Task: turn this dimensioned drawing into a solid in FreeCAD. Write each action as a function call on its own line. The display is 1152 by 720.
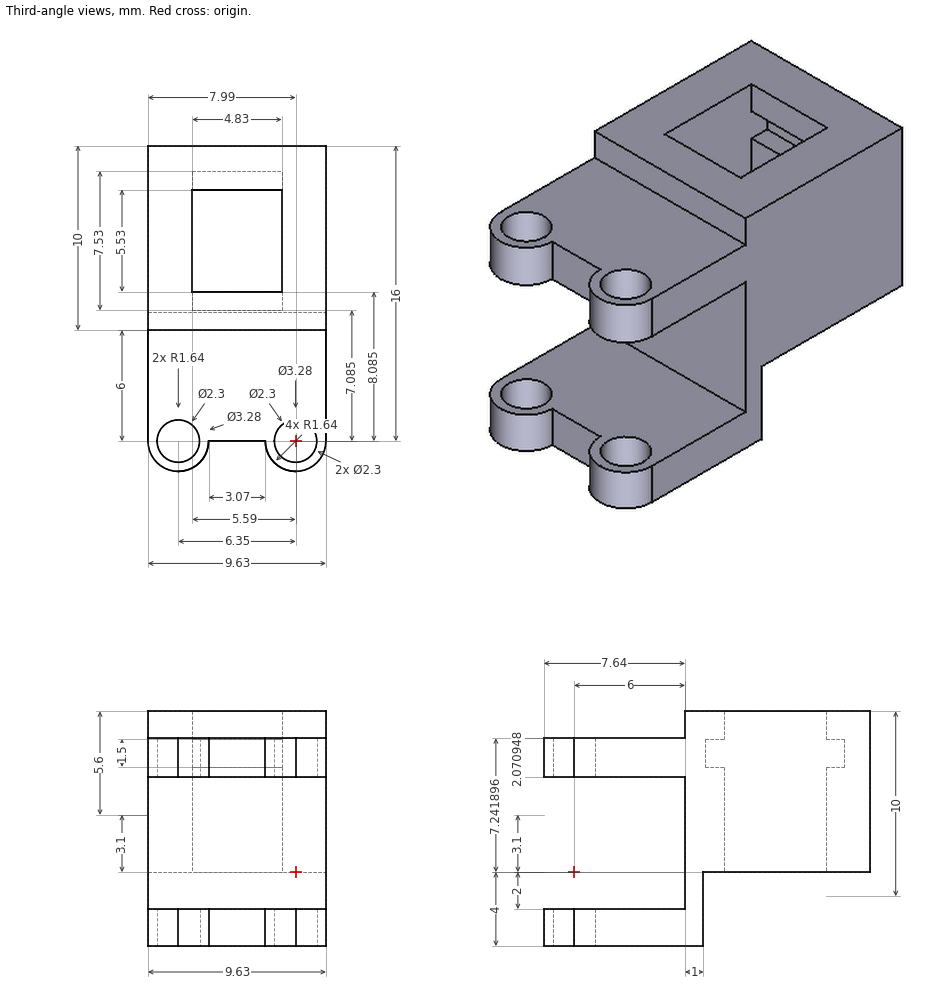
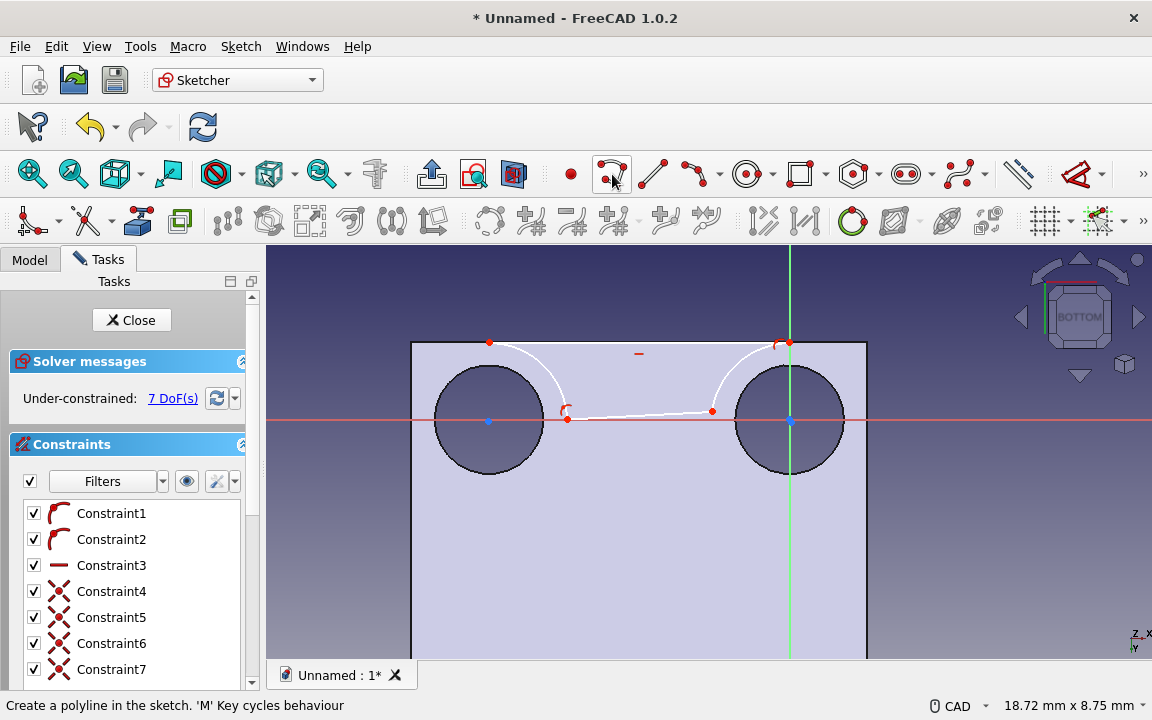
click(867, 420)
click(867, 342)
click(790, 343)
right_click(867, 342)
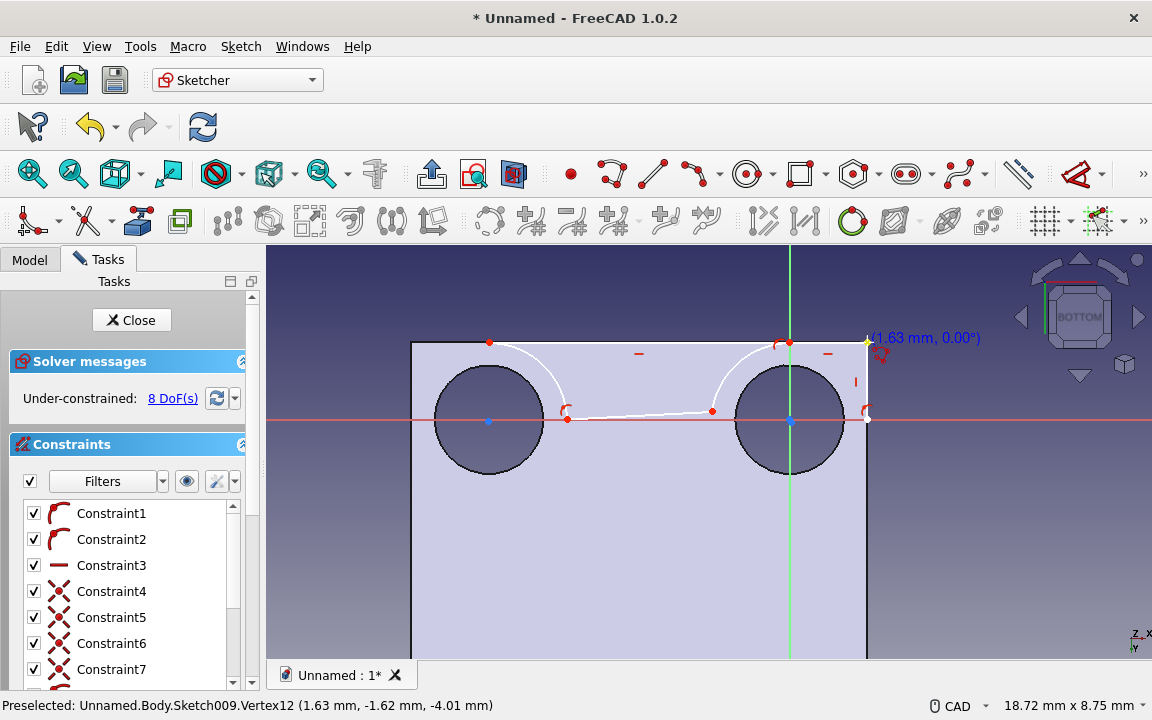
click(694, 174)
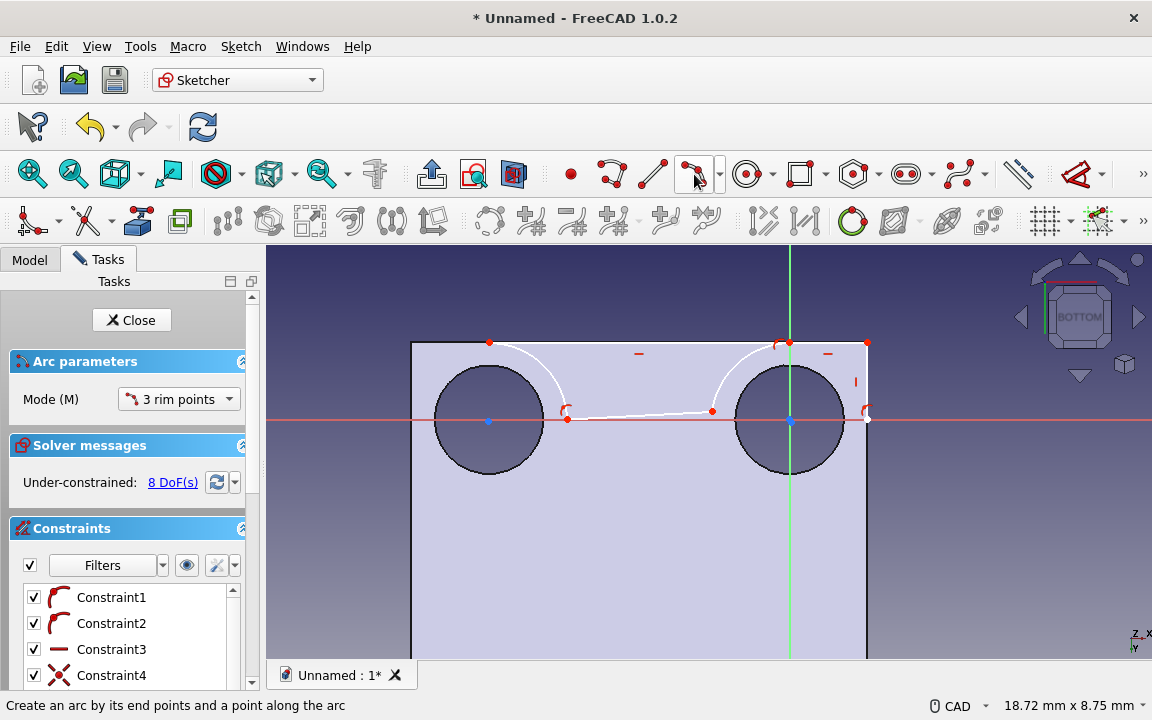
click(790, 343)
click(867, 420)
click(845, 365)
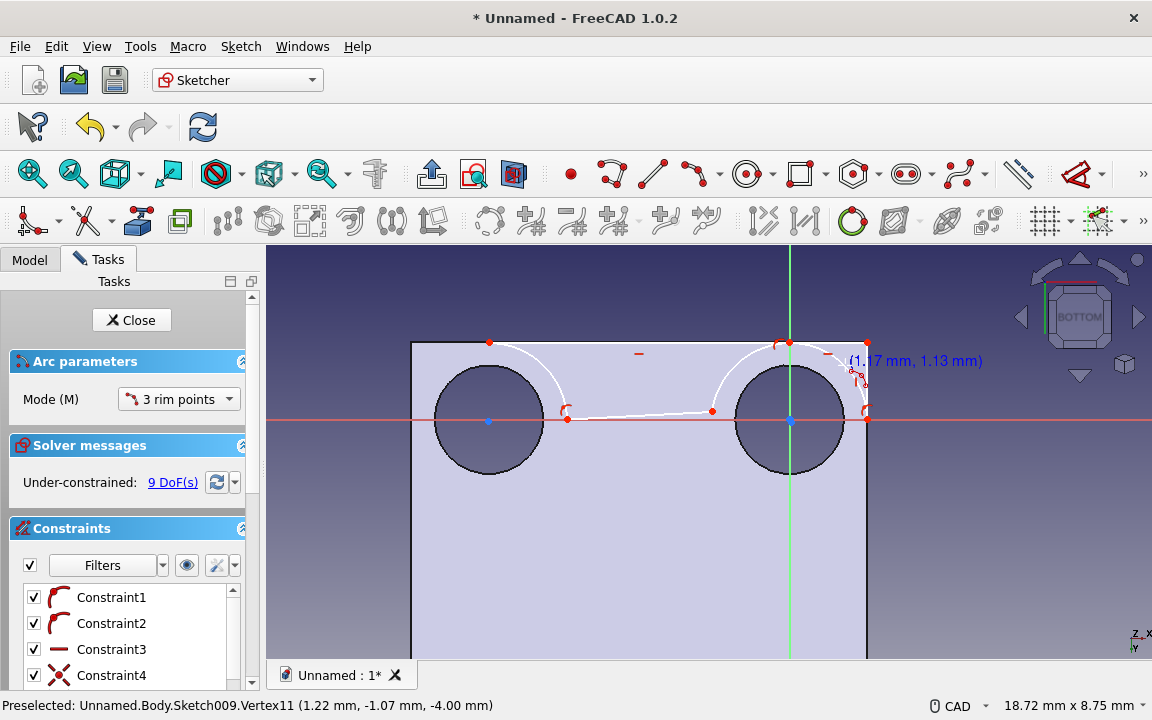
click(612, 174)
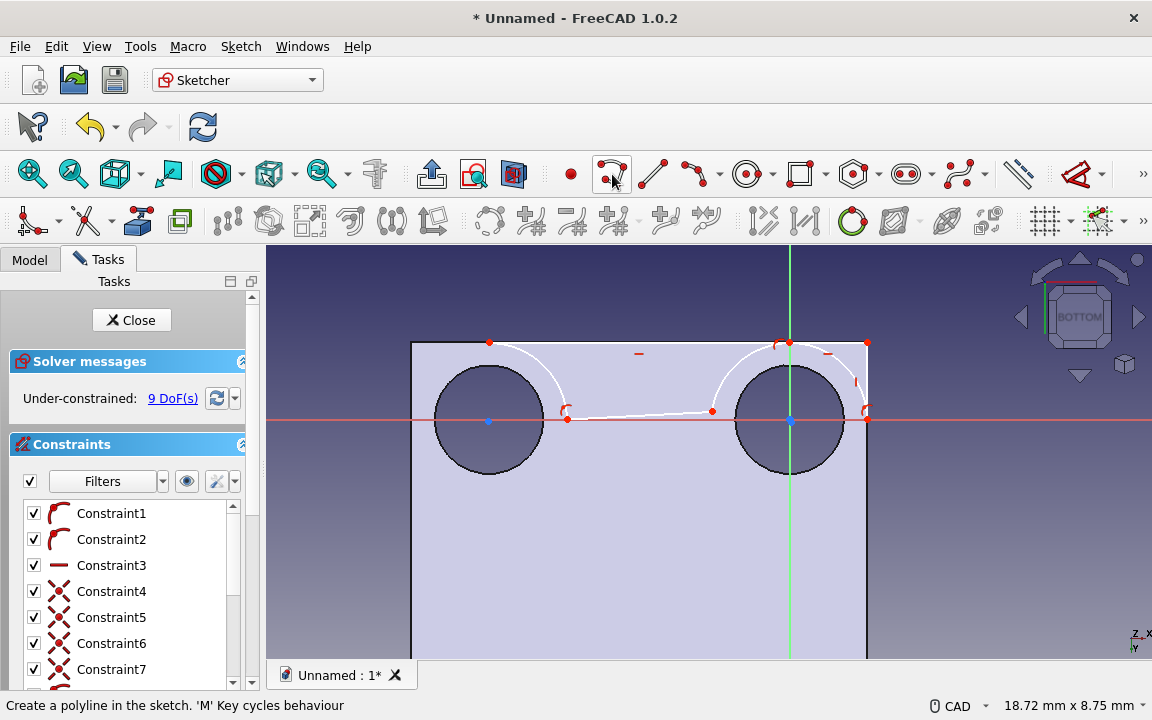
click(489, 343)
click(411, 342)
click(411, 420)
right_click(411, 420)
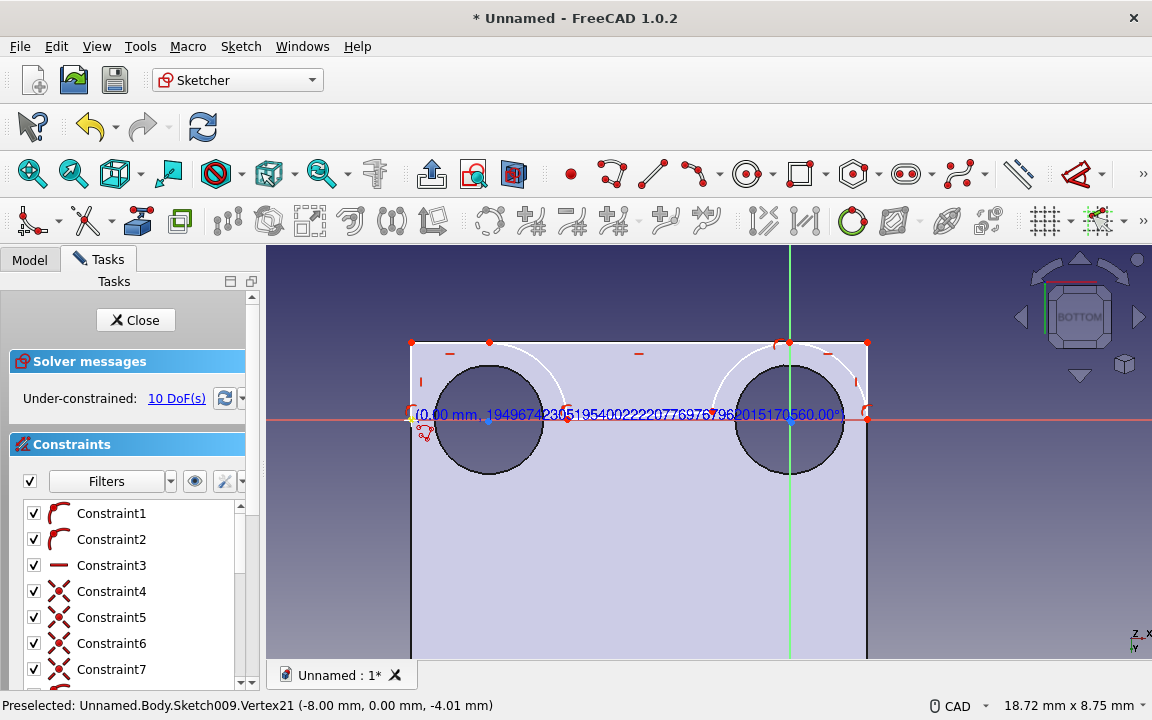
click(694, 174)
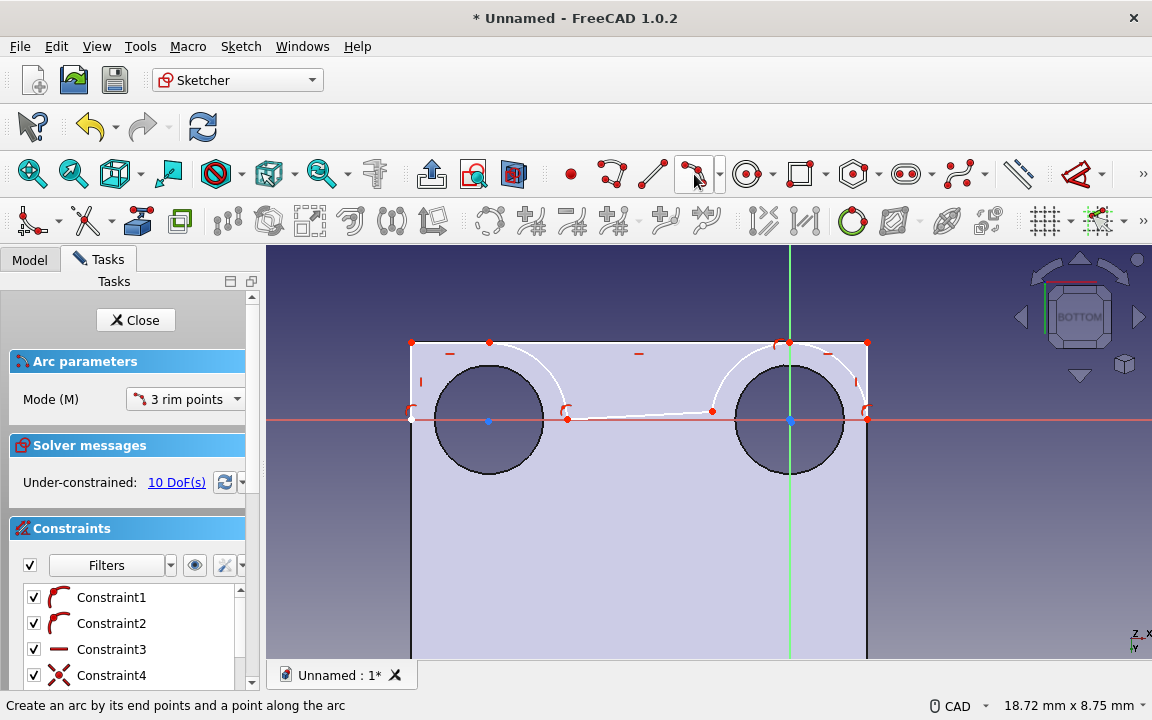
click(411, 420)
click(489, 343)
click(434, 365)
key(Escape)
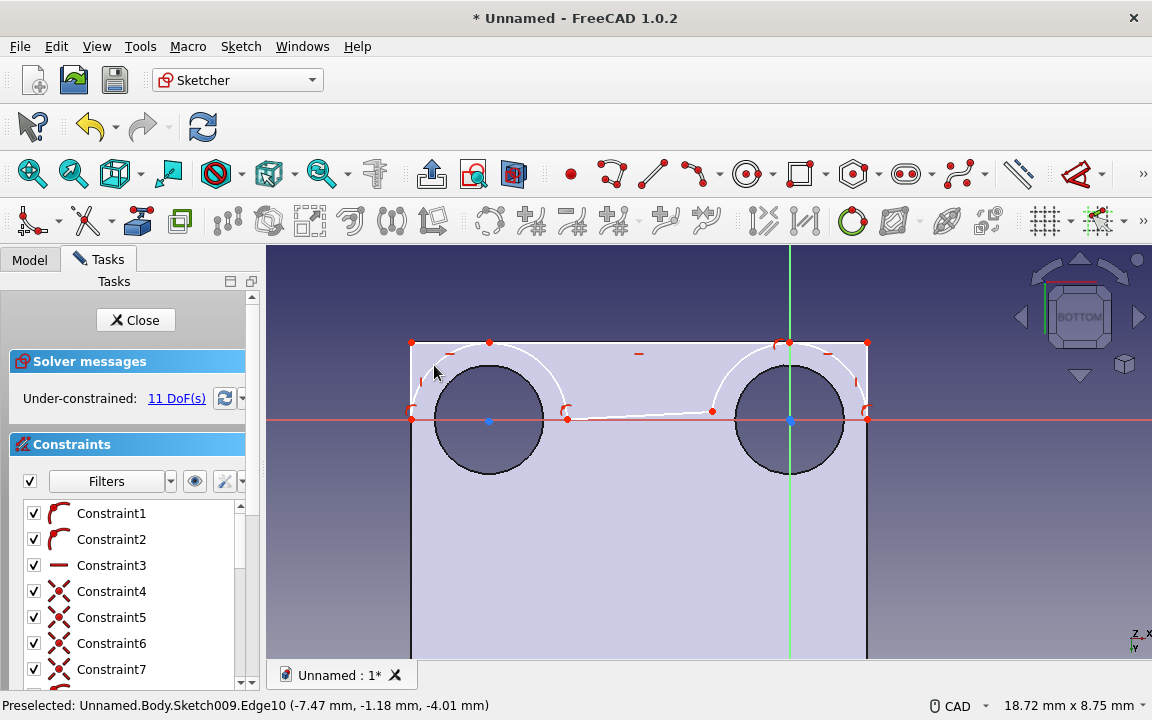
click(699, 343)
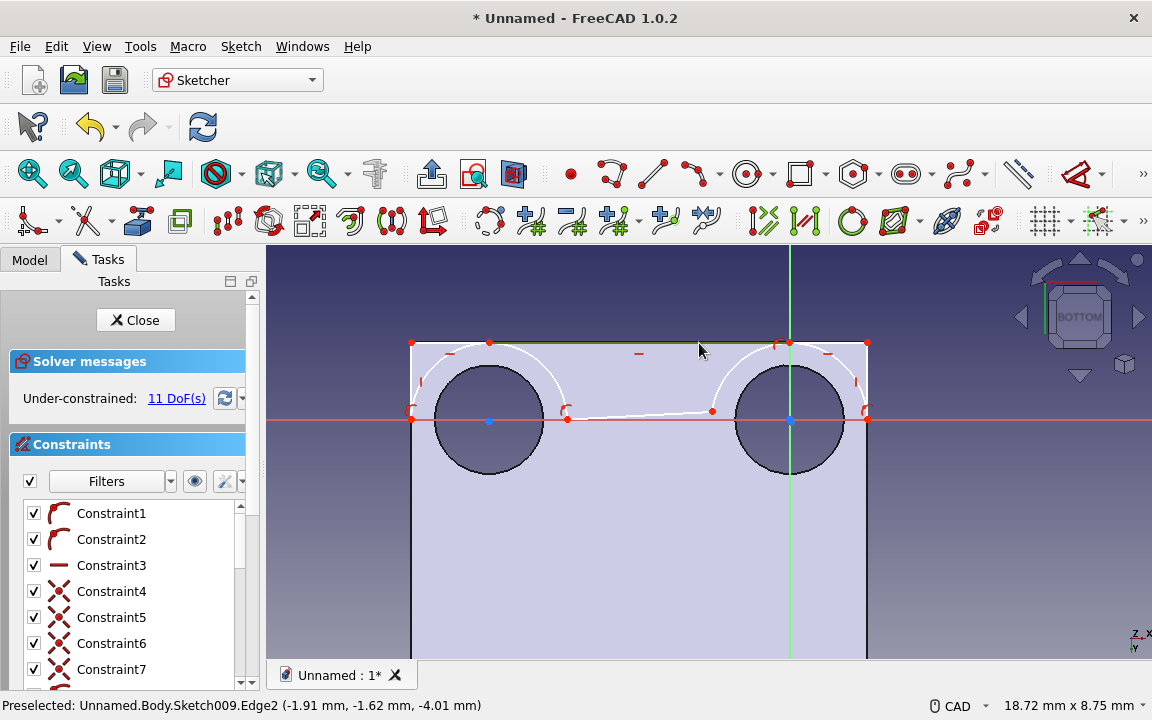
click(723, 380)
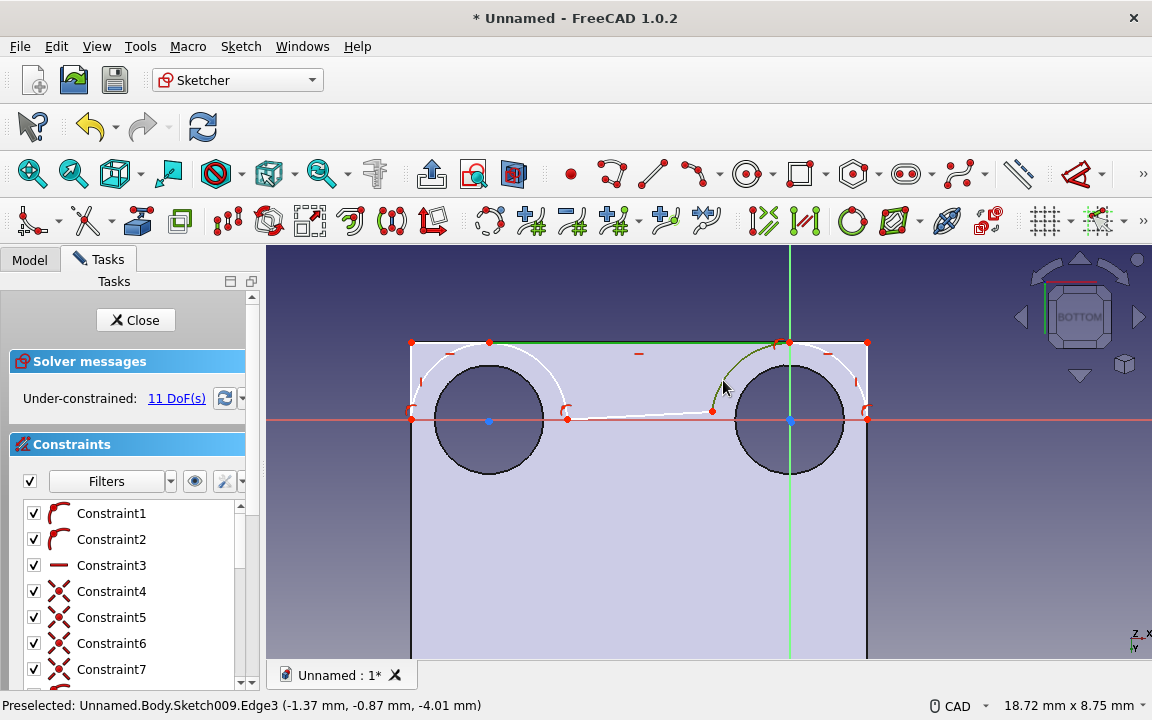
key(t)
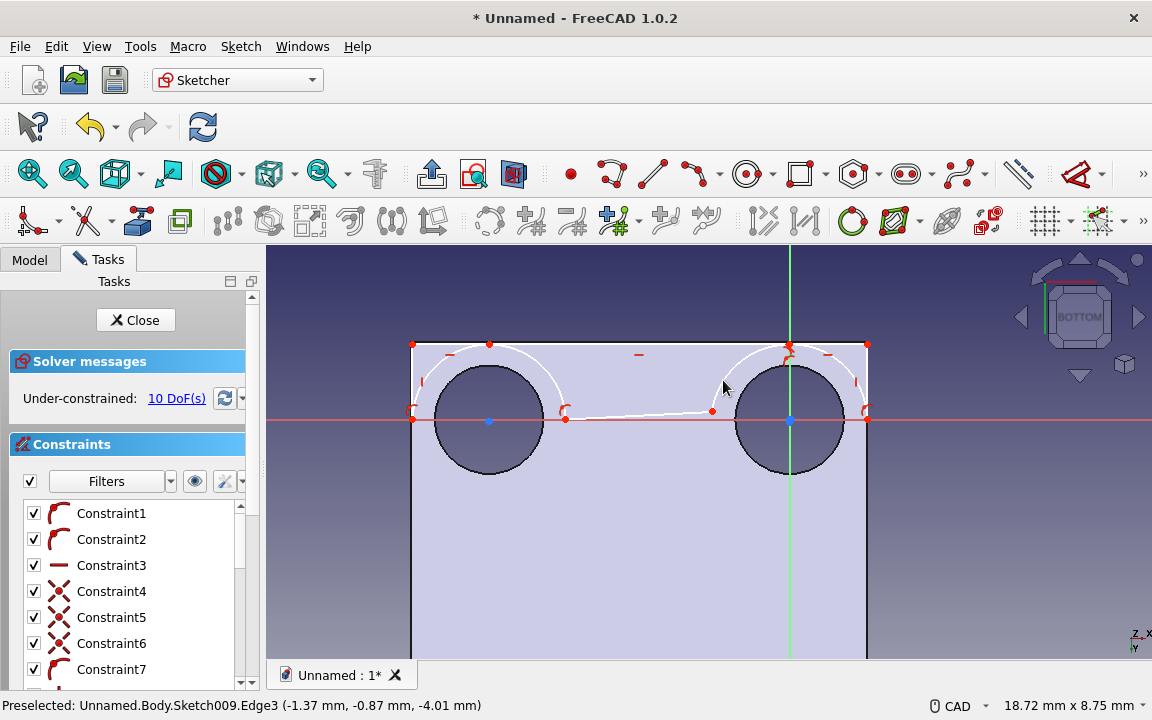
click(699, 344)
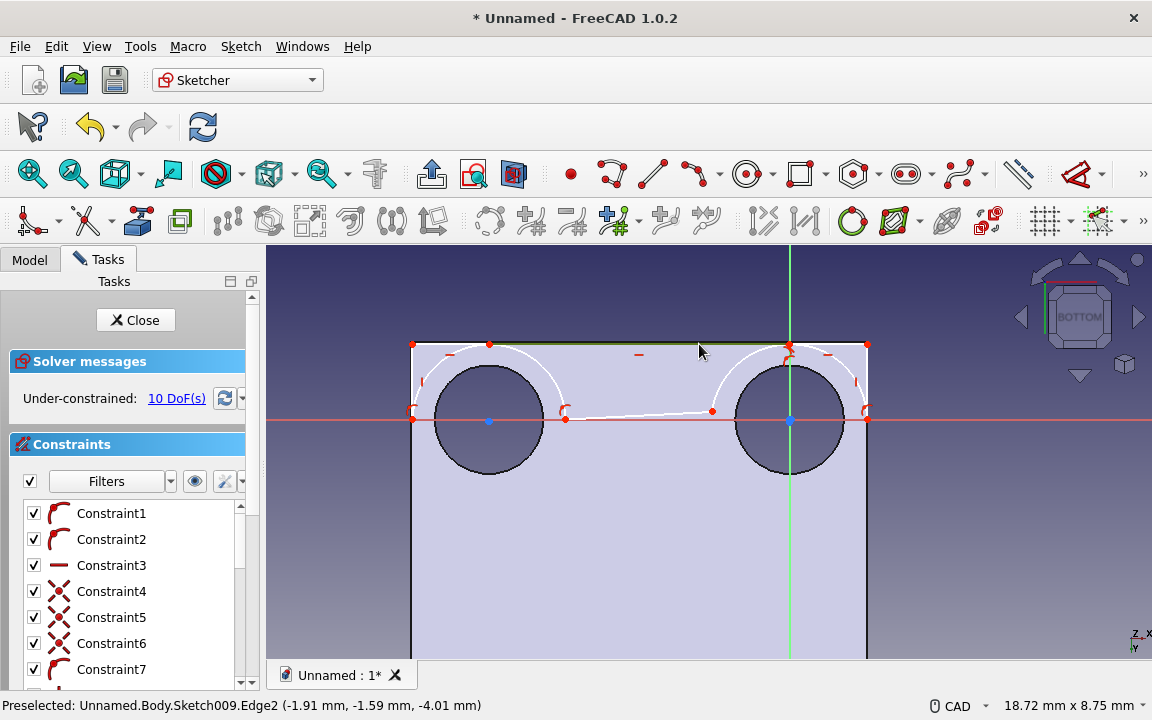
click(557, 385)